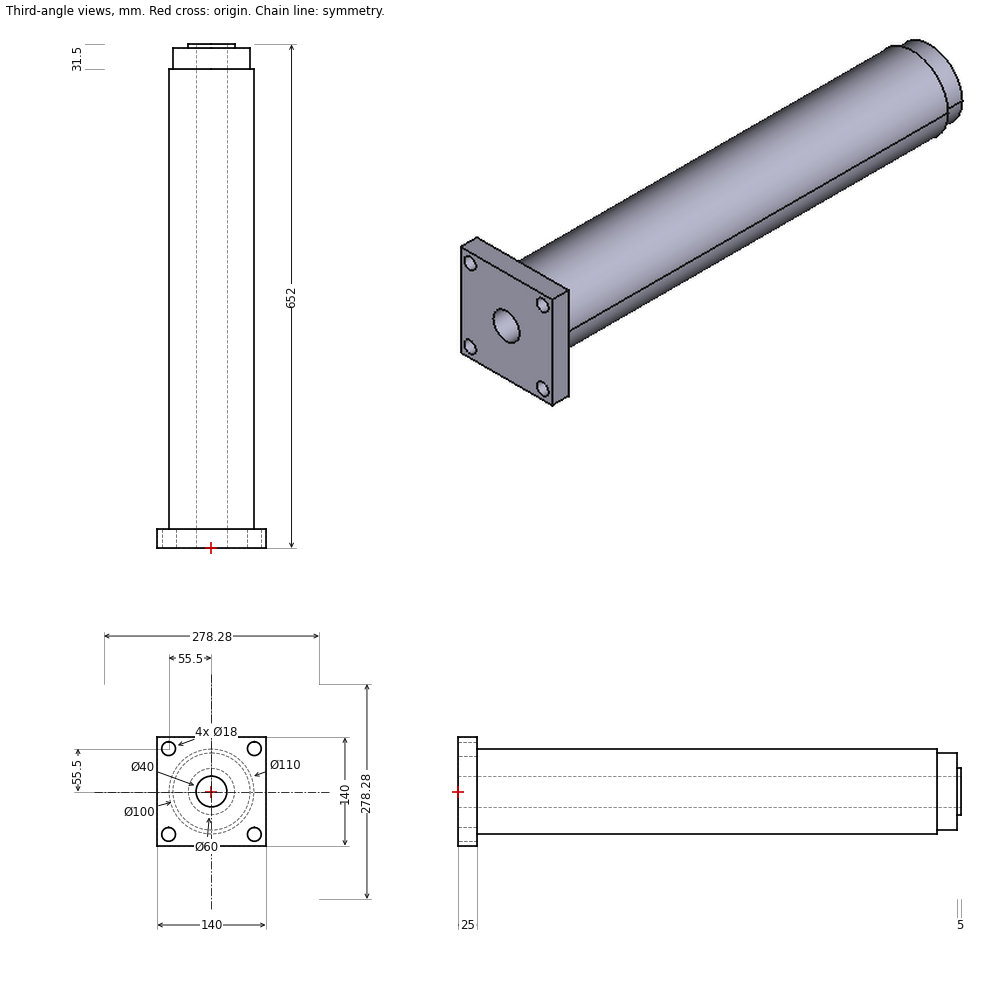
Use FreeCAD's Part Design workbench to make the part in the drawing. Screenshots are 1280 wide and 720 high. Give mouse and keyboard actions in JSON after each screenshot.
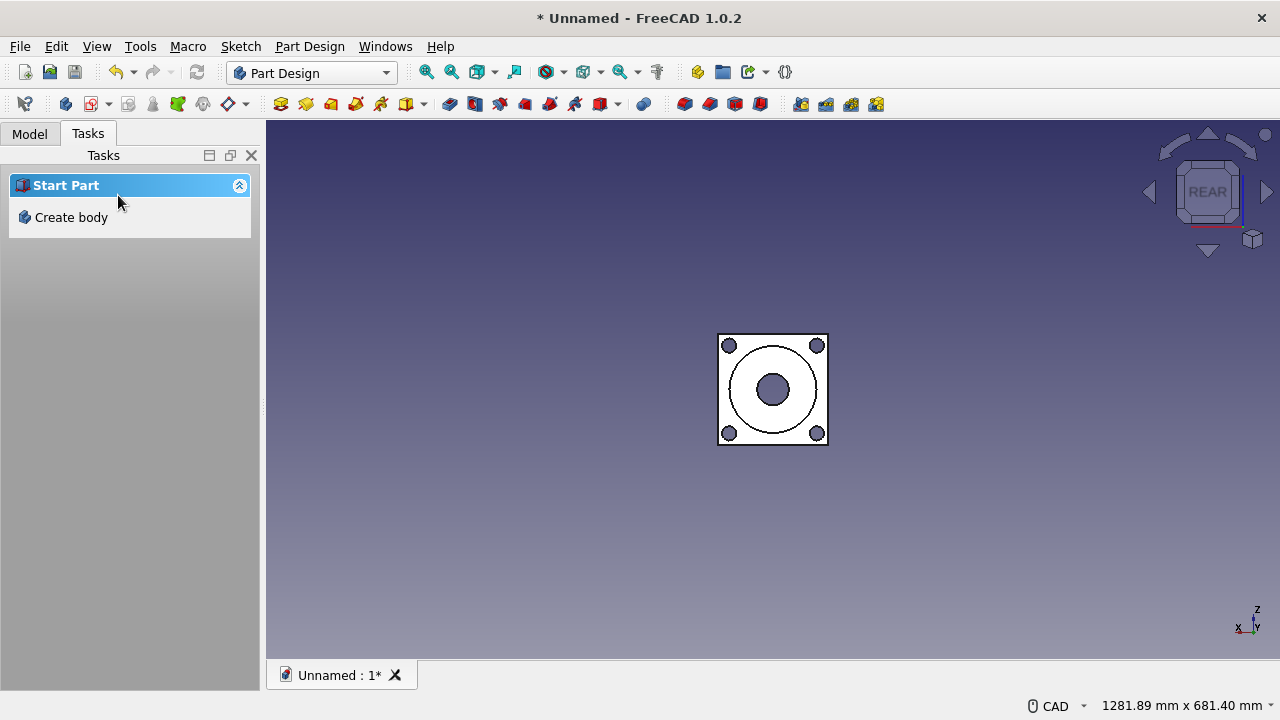
{"action": "left_click", "coordinate": [785, 413]}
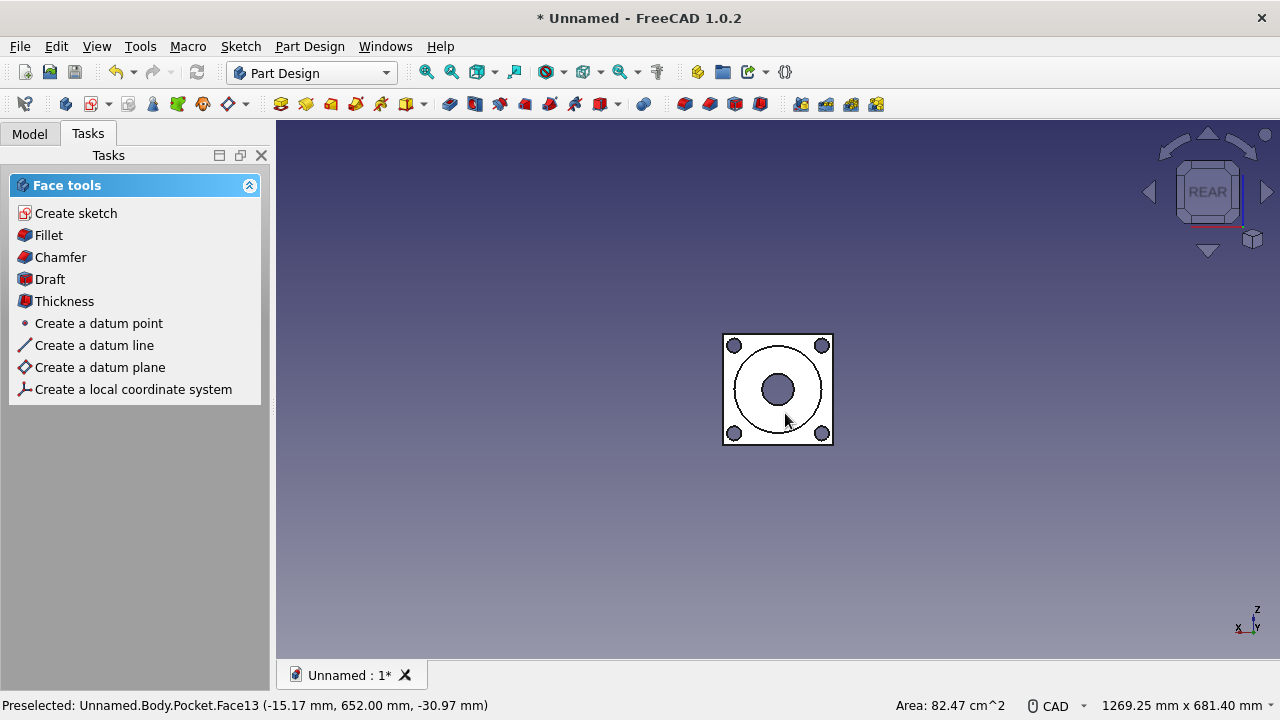
{"action": "left_click", "coordinate": [90, 104]}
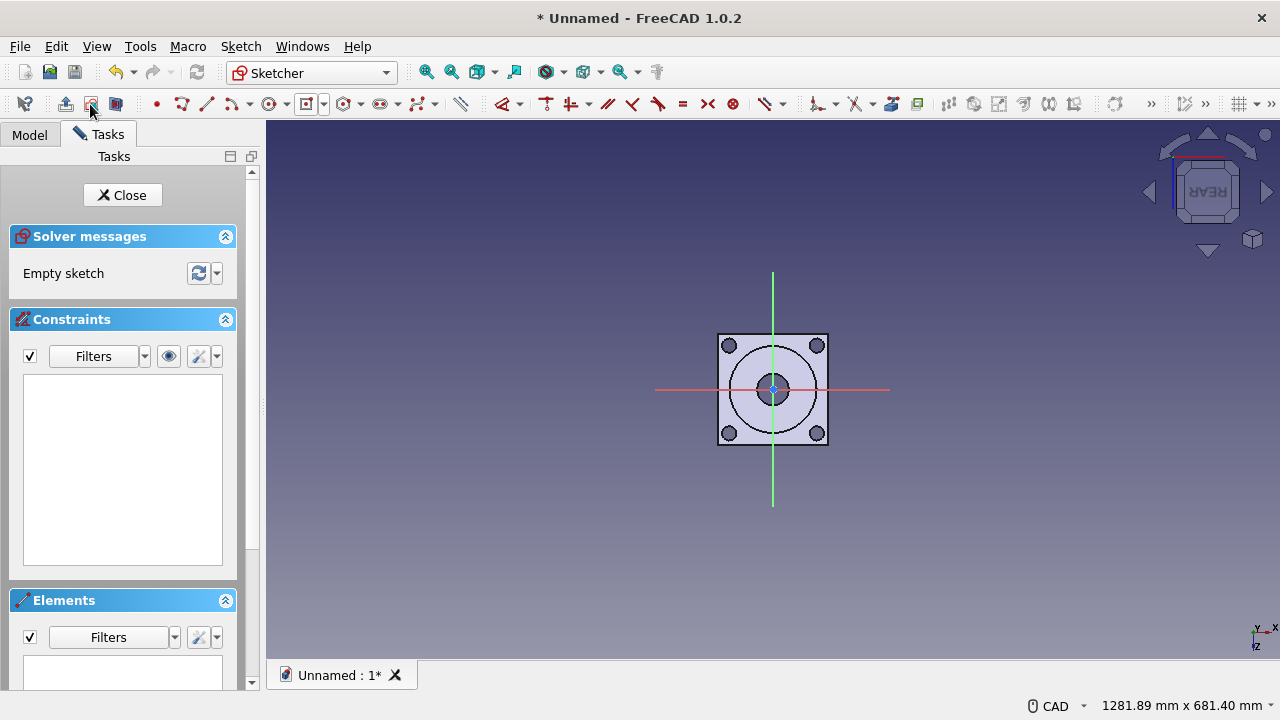
{"action": "scroll", "coordinate": [912, 389], "scroll_direction": "up", "scroll_amount": 2}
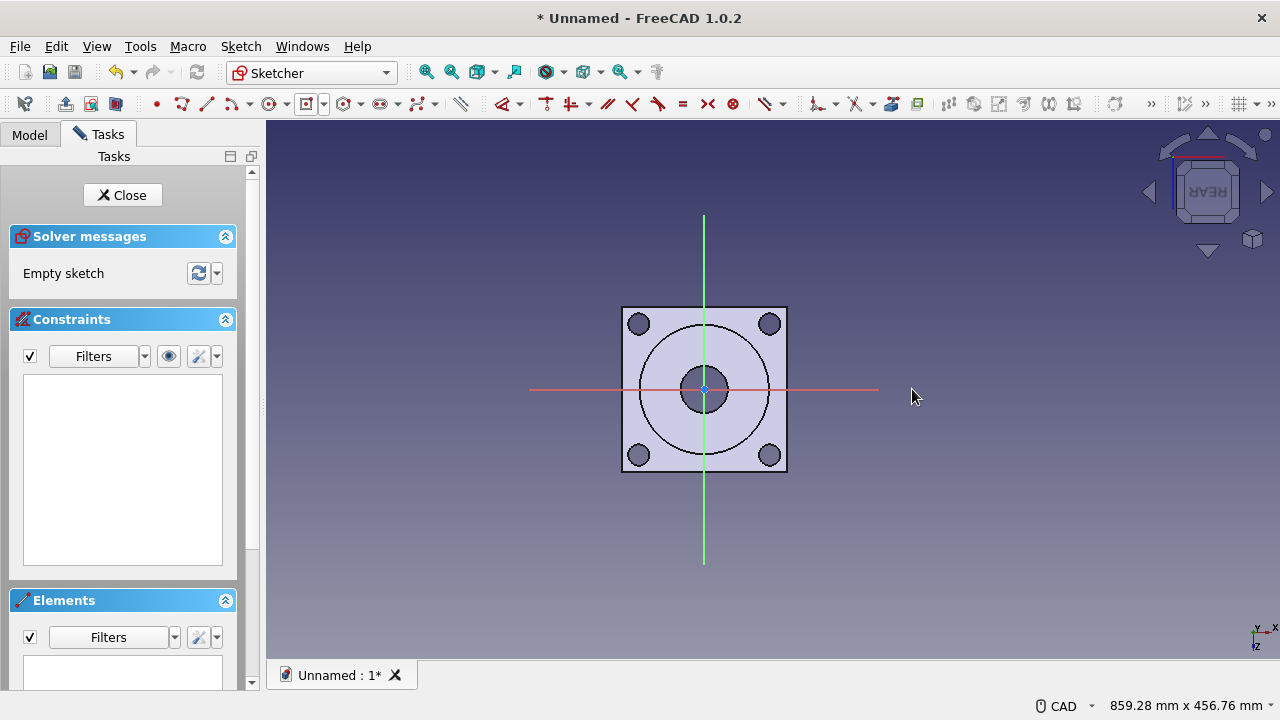
{"action": "left_click", "coordinate": [306, 104]}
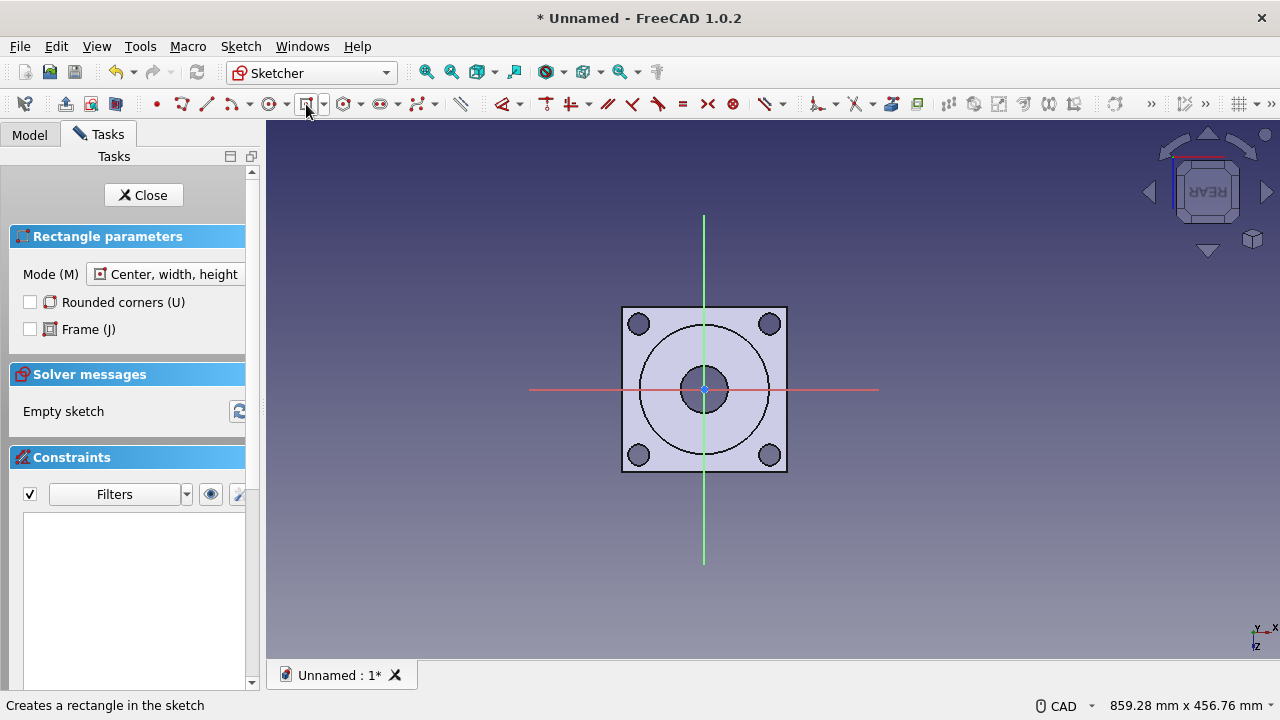
{"action": "left_click", "coordinate": [704, 389]}
{"action": "mouse_move", "coordinate": [869, 225]}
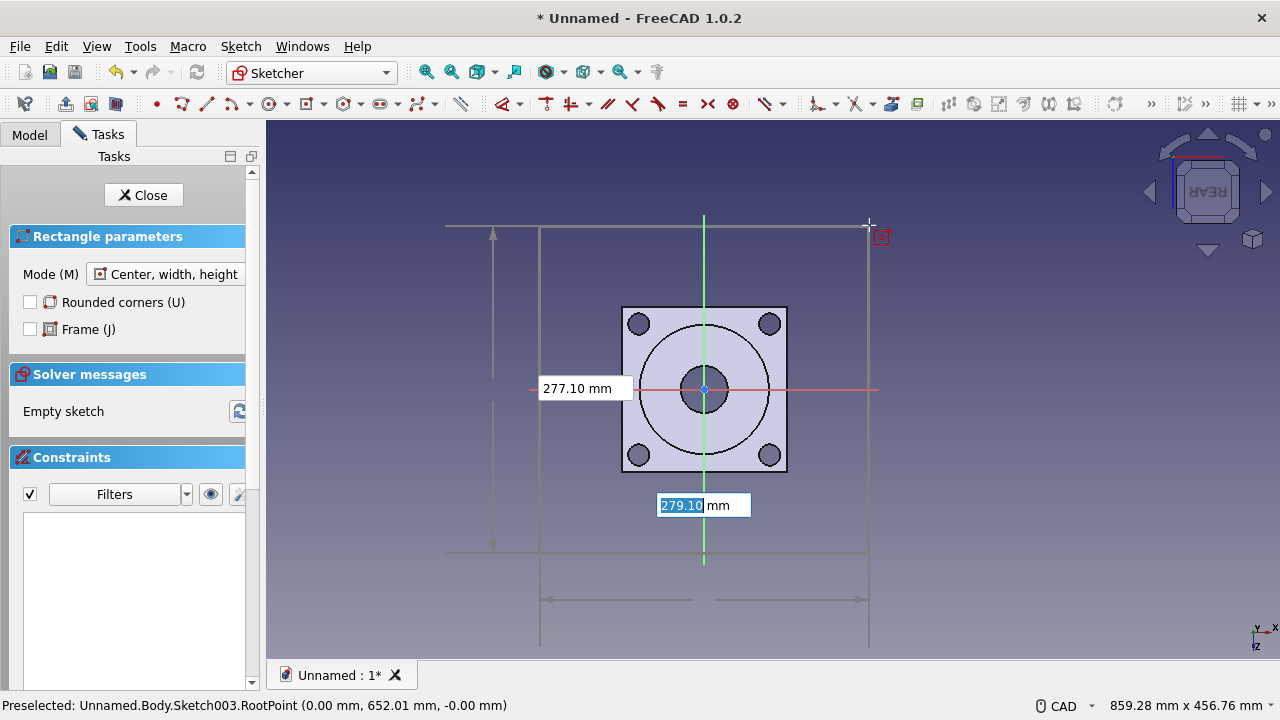
{"action": "type", "text": "278.28"}
{"action": "key", "text": "Tab"}
{"action": "type", "text": "278.28"}
{"action": "key", "text": "Return"}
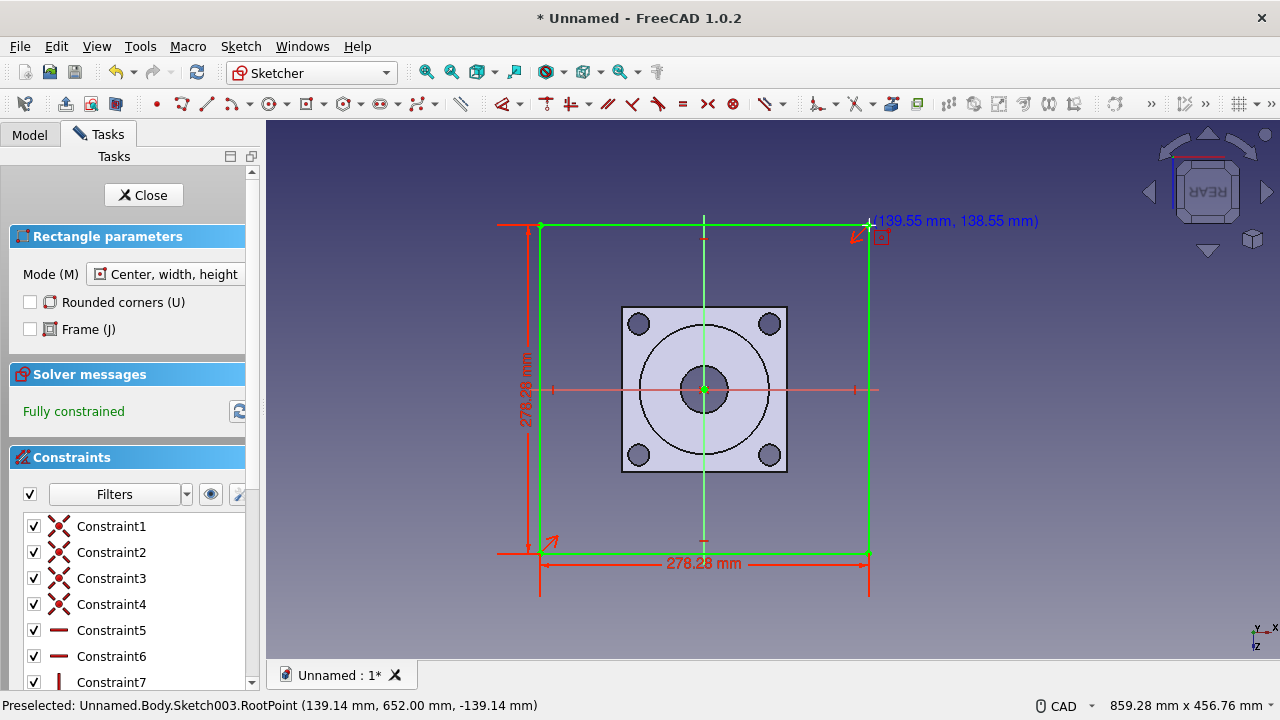
{"action": "left_click", "coordinate": [268, 104]}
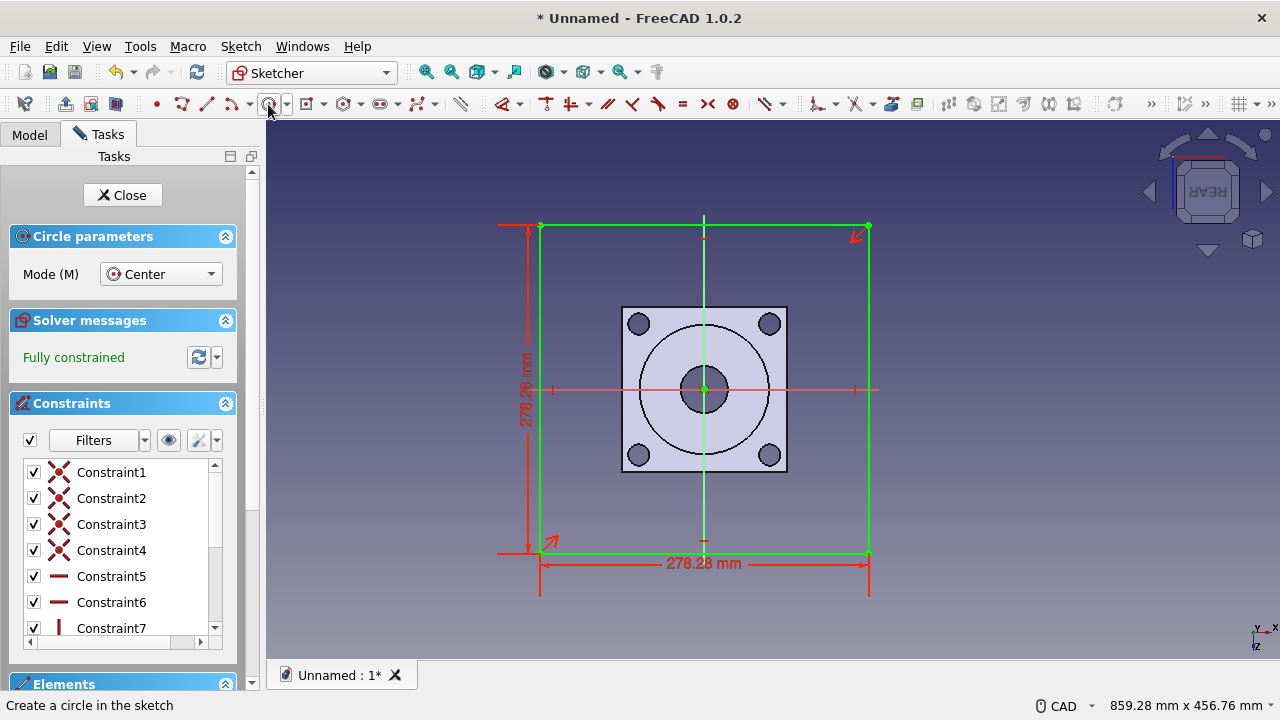
{"action": "left_click", "coordinate": [704, 389]}
{"action": "mouse_move", "coordinate": [729, 364]}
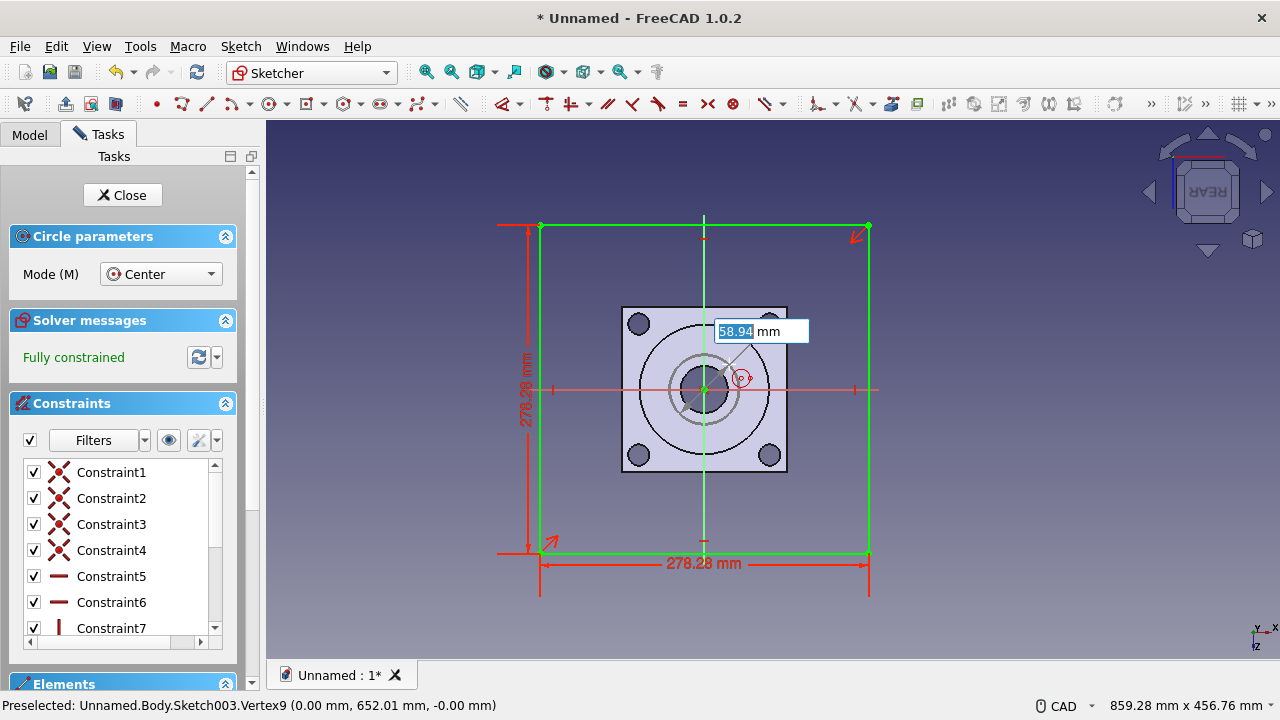
{"action": "type", "text": "60"}
{"action": "key", "text": "Return"}
{"action": "key", "text": "Escape"}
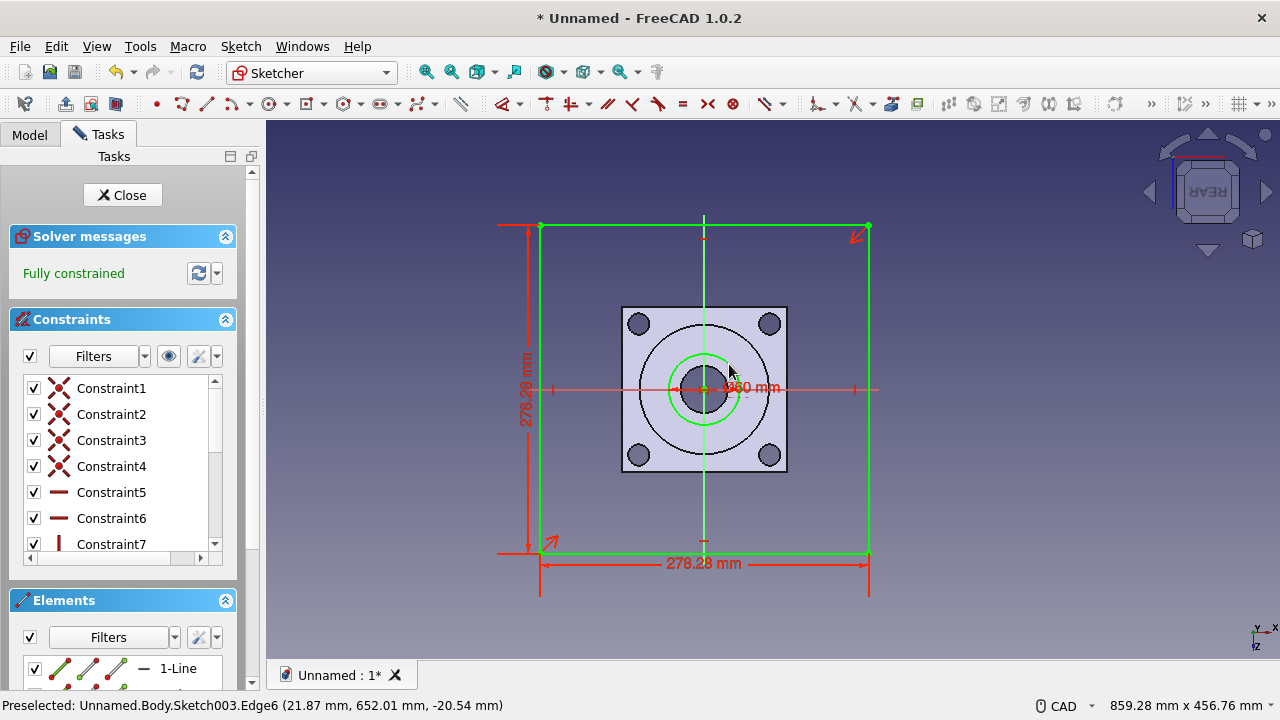
{"action": "left_click", "coordinate": [123, 195]}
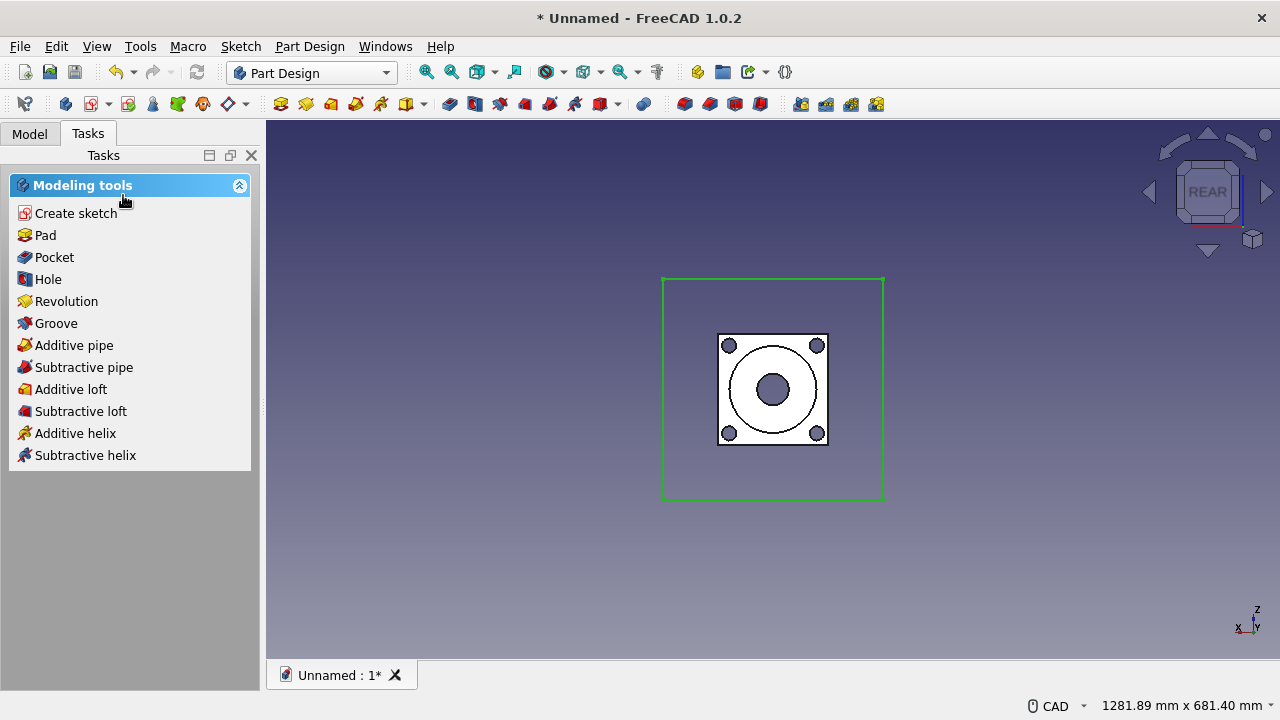
{"action": "left_click", "coordinate": [450, 104]}